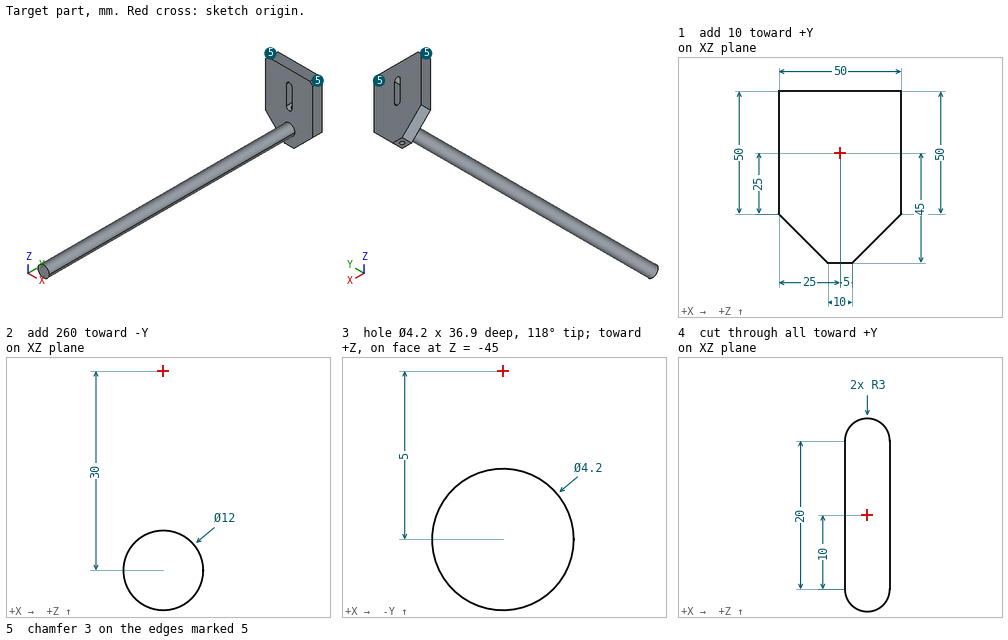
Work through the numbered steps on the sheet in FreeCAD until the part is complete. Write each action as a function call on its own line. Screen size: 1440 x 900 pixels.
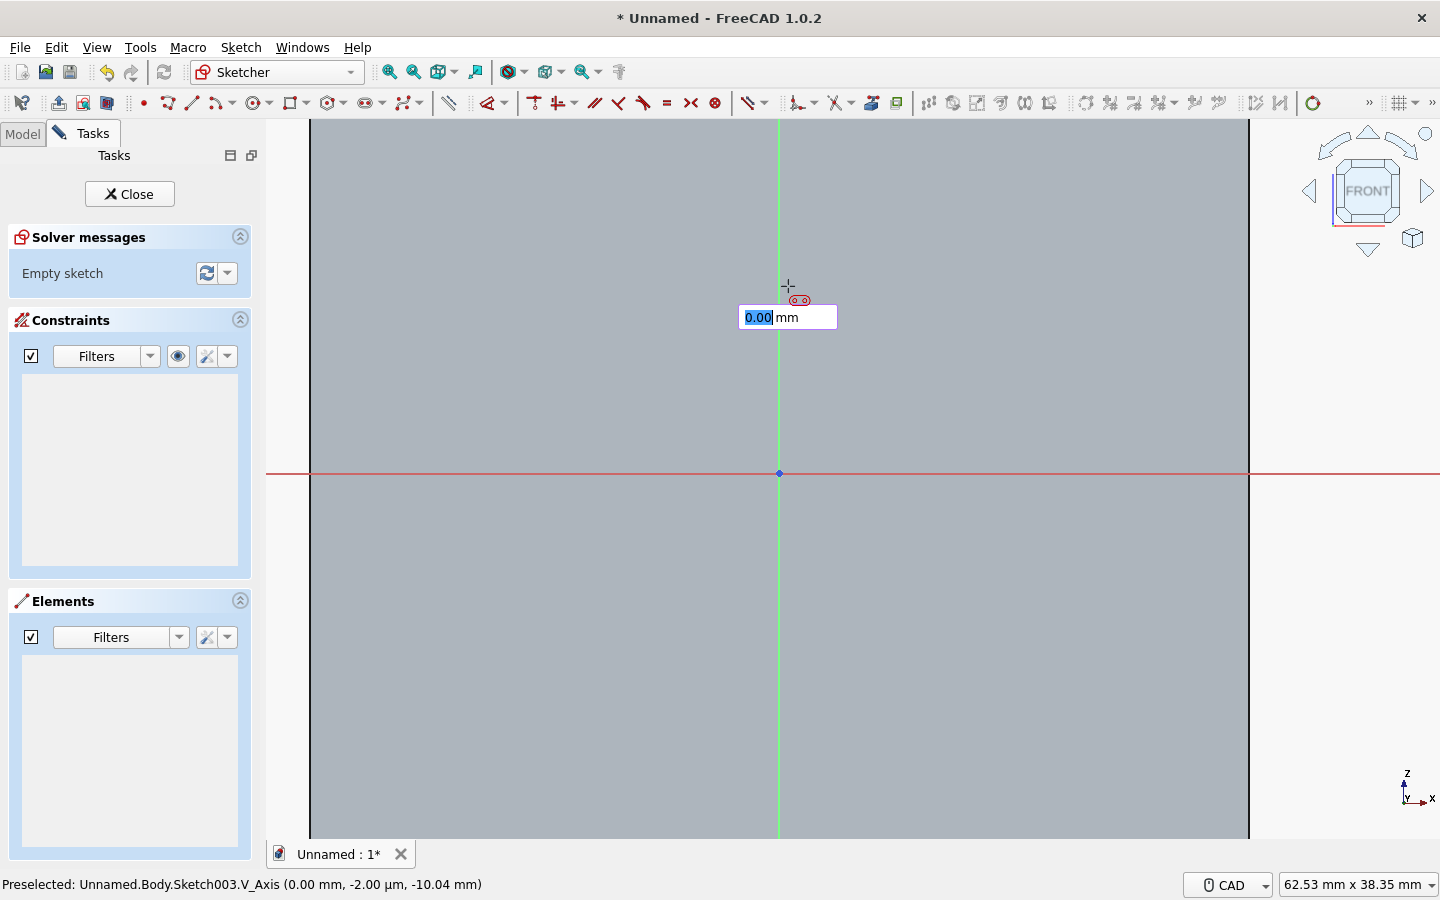
click(836, 530)
key(Escape)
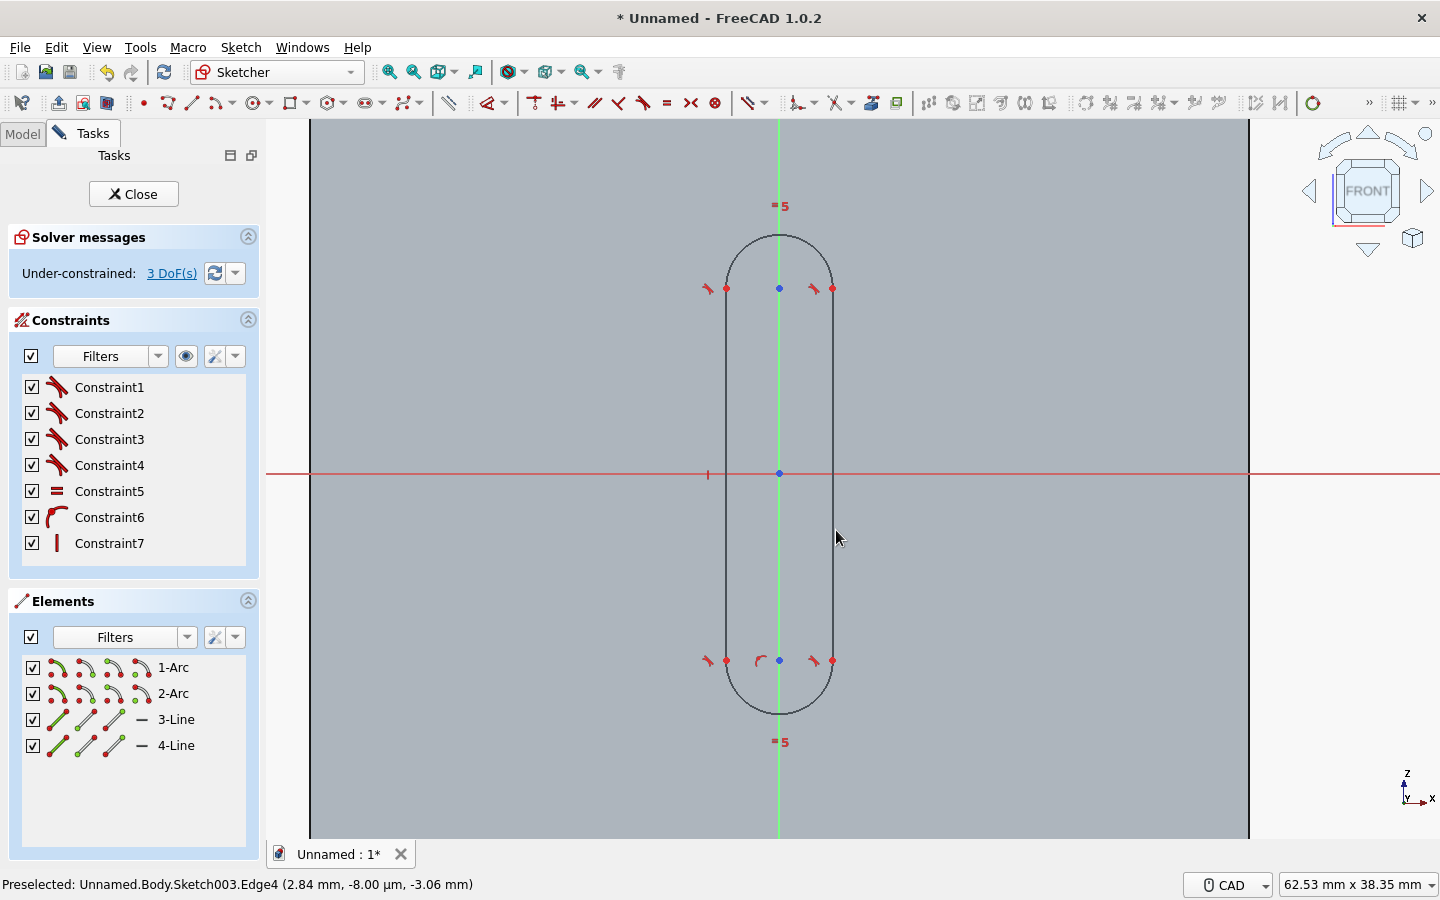
click(488, 104)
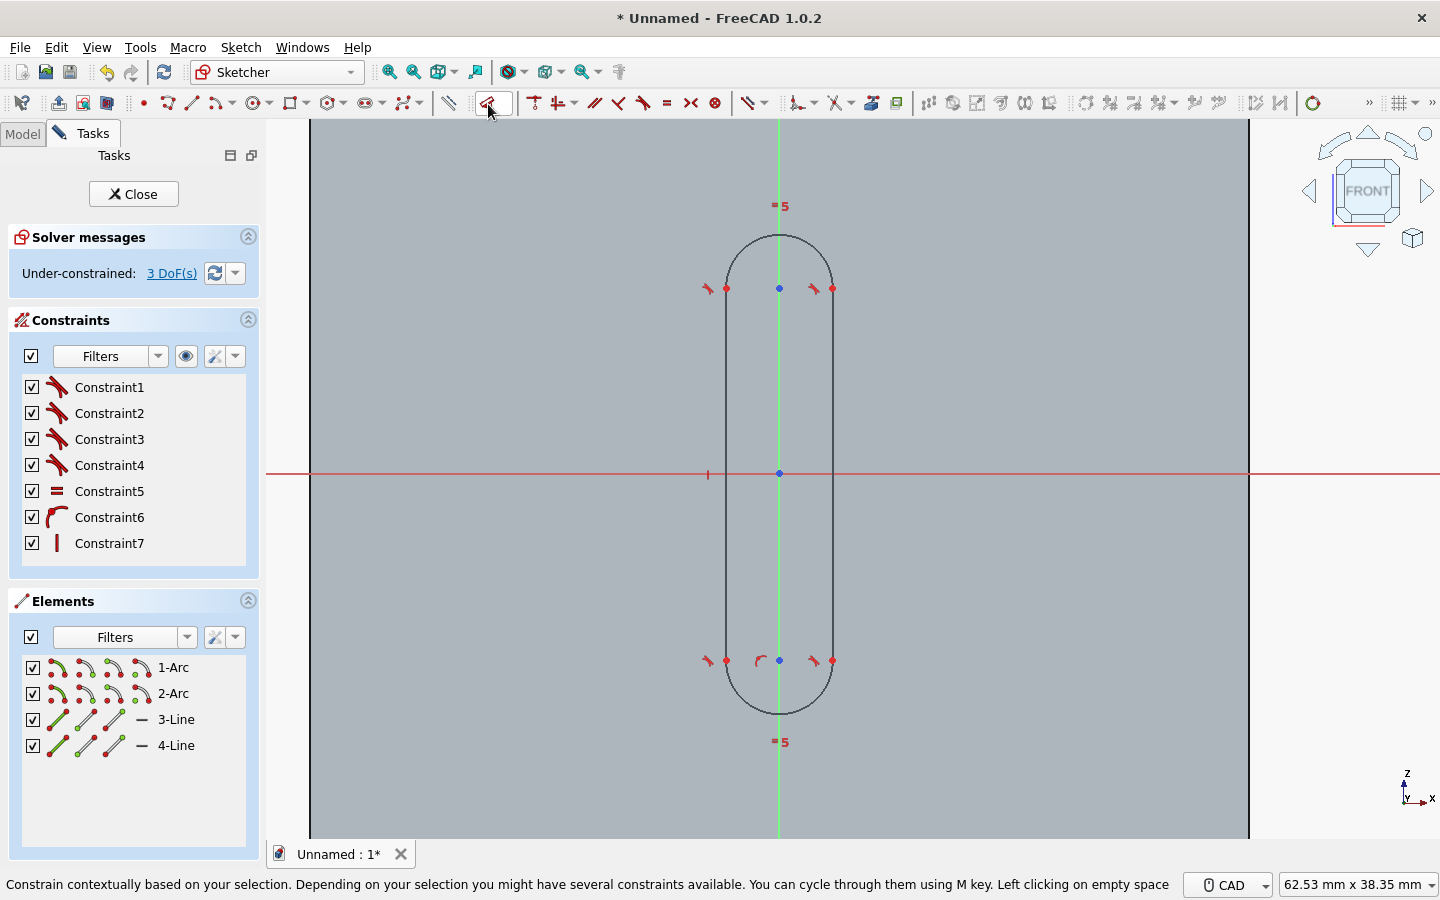
click(748, 704)
click(729, 730)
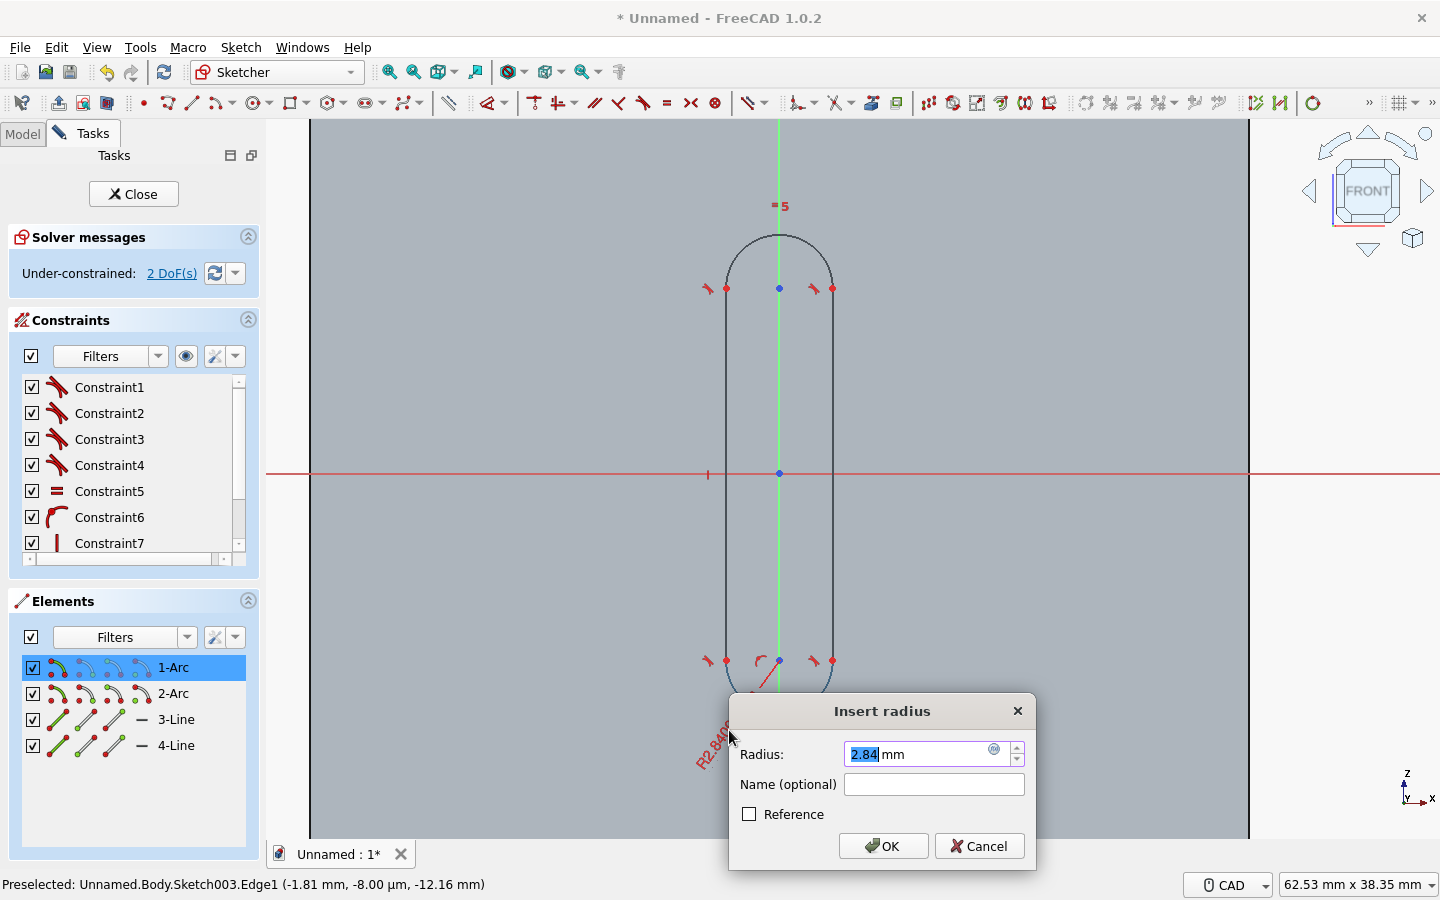
text(3)
key(Return)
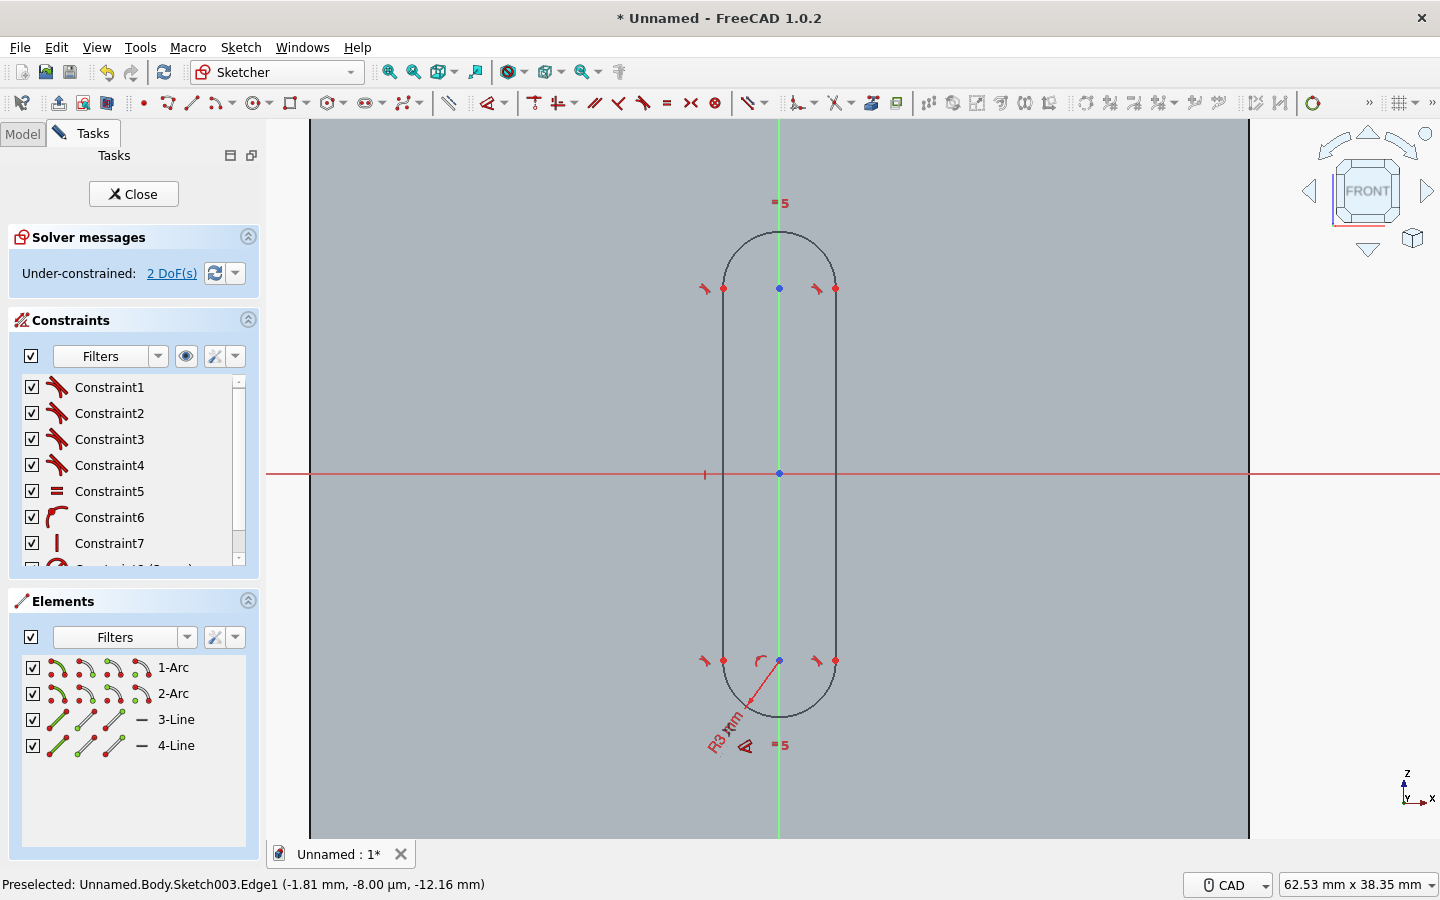
click(723, 549)
click(689, 389)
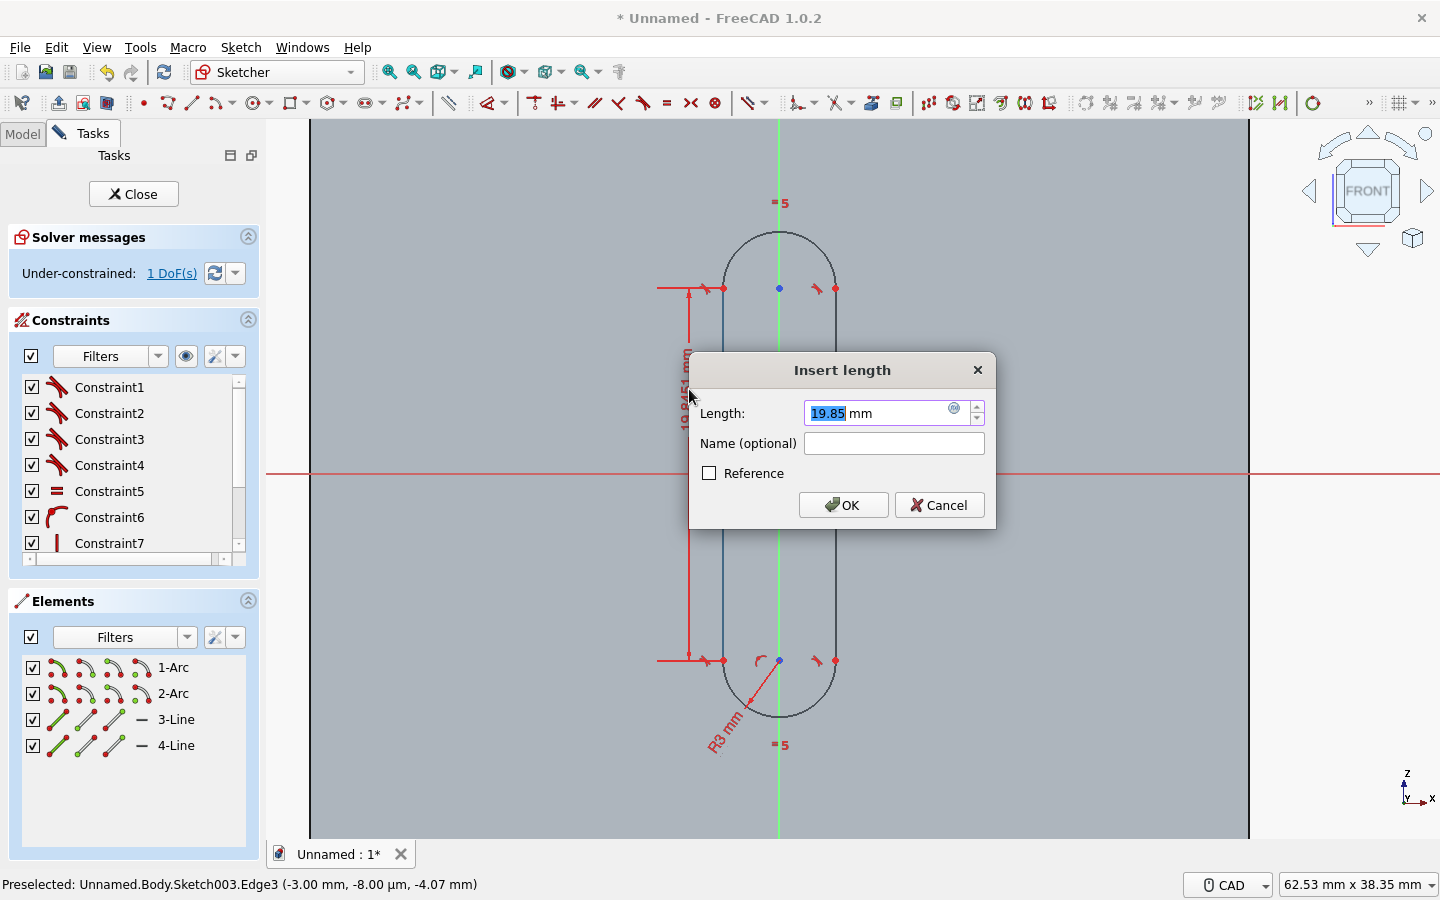
text(20)
key(Return)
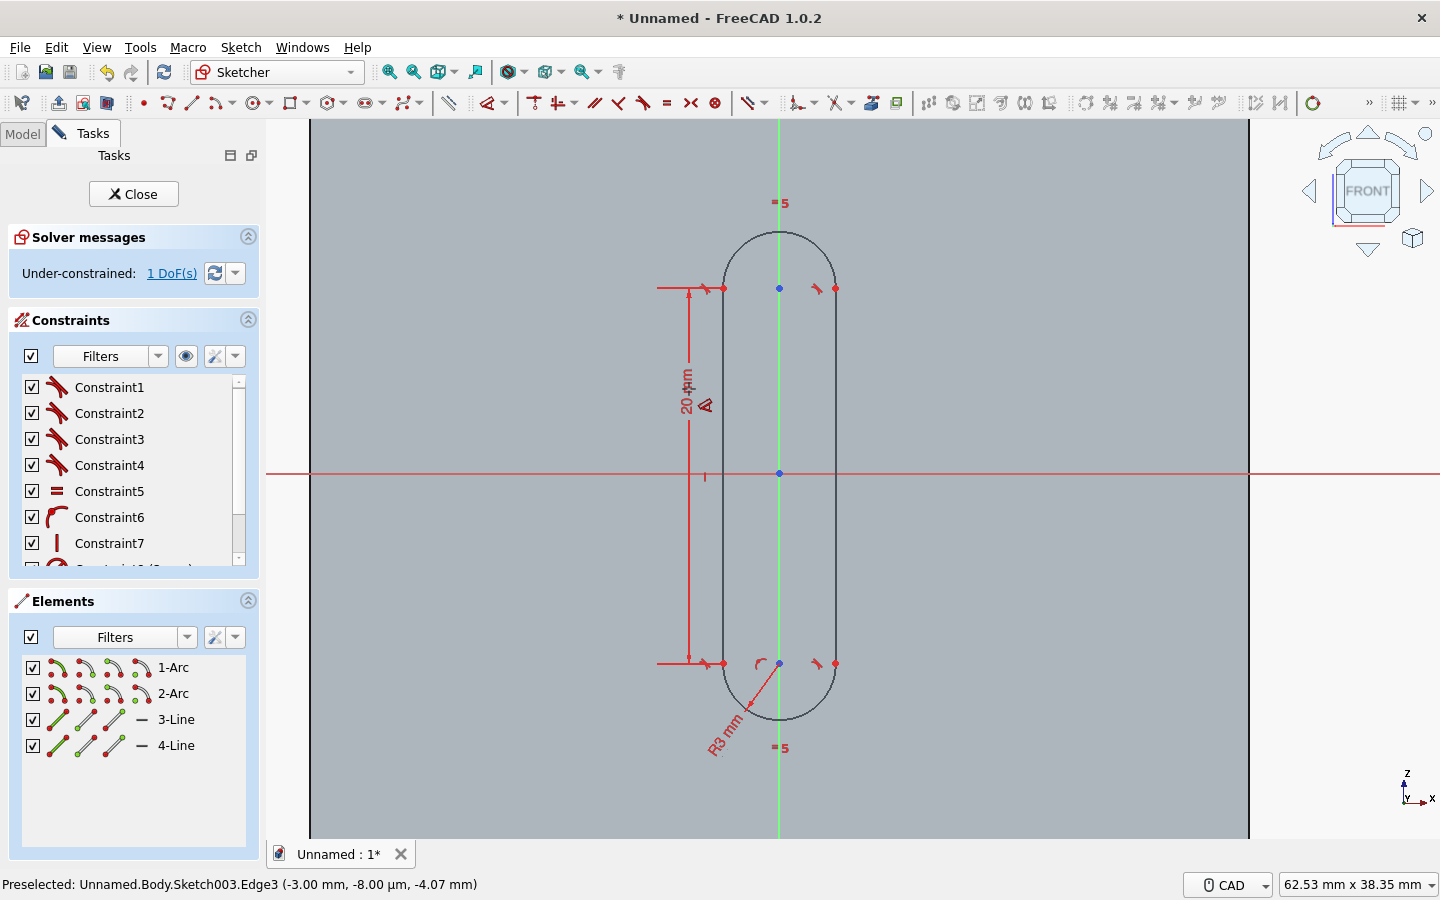
click(723, 664)
click(689, 569)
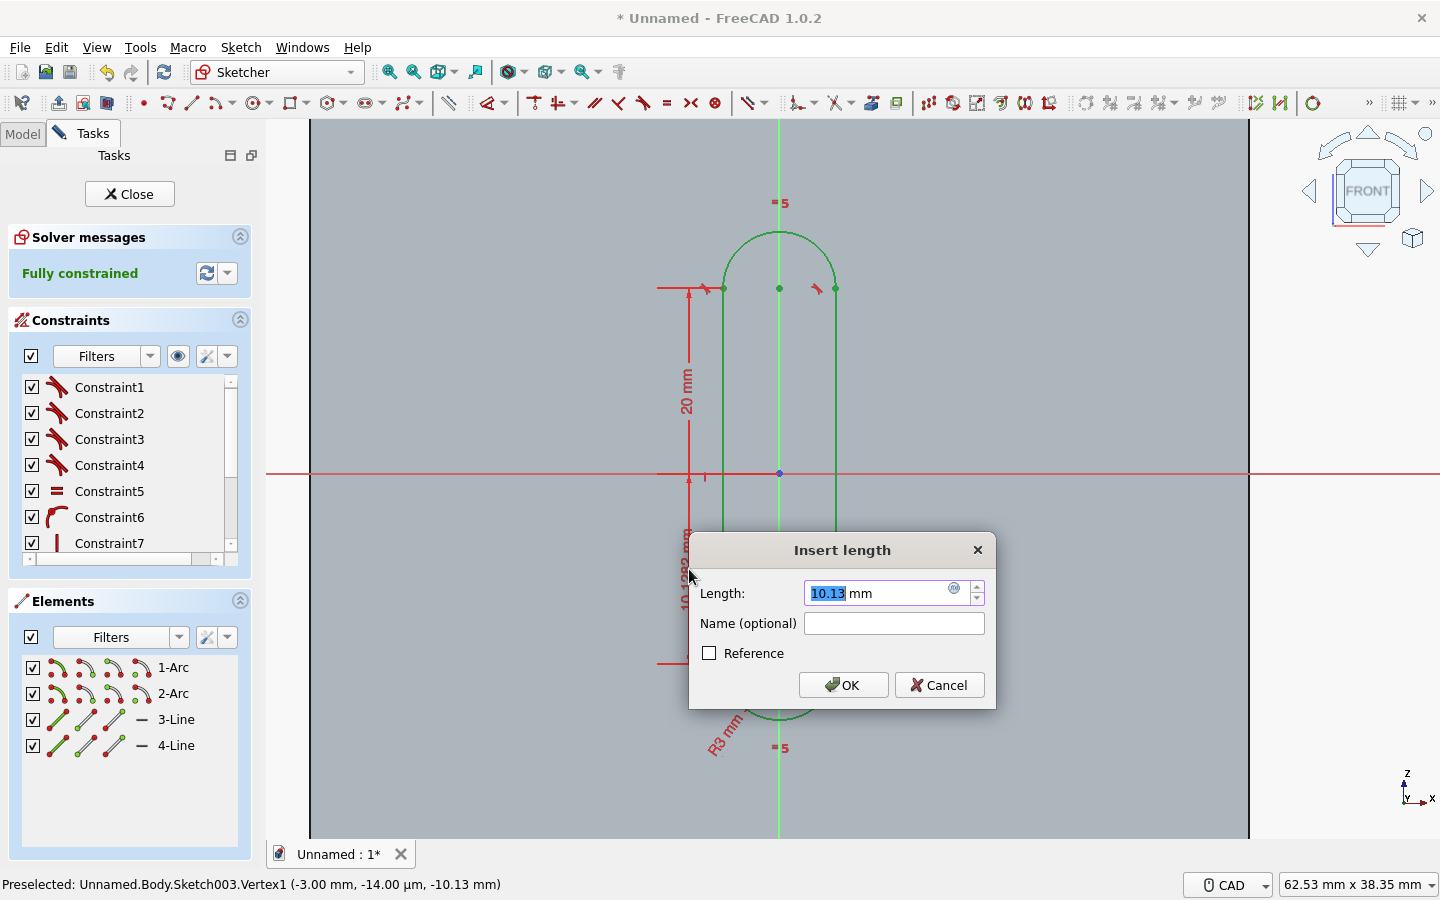
text(10)
key(Return)
key(Escape)